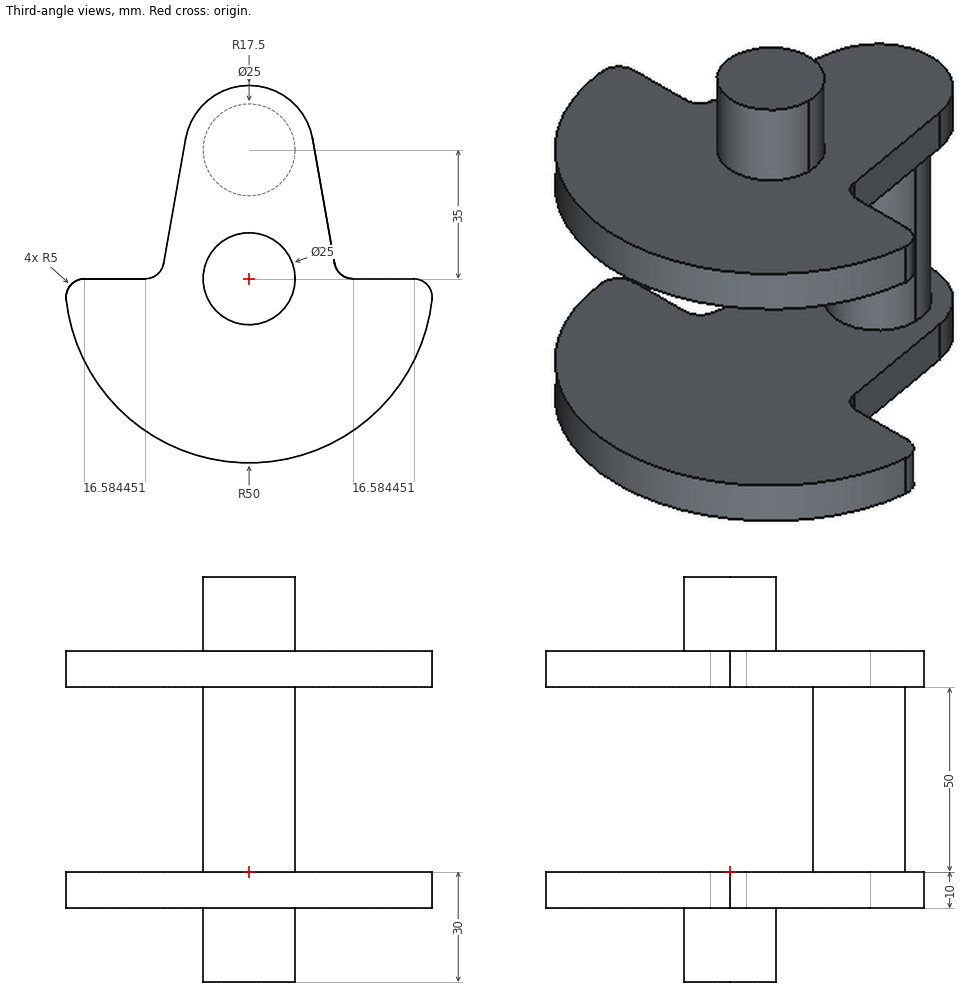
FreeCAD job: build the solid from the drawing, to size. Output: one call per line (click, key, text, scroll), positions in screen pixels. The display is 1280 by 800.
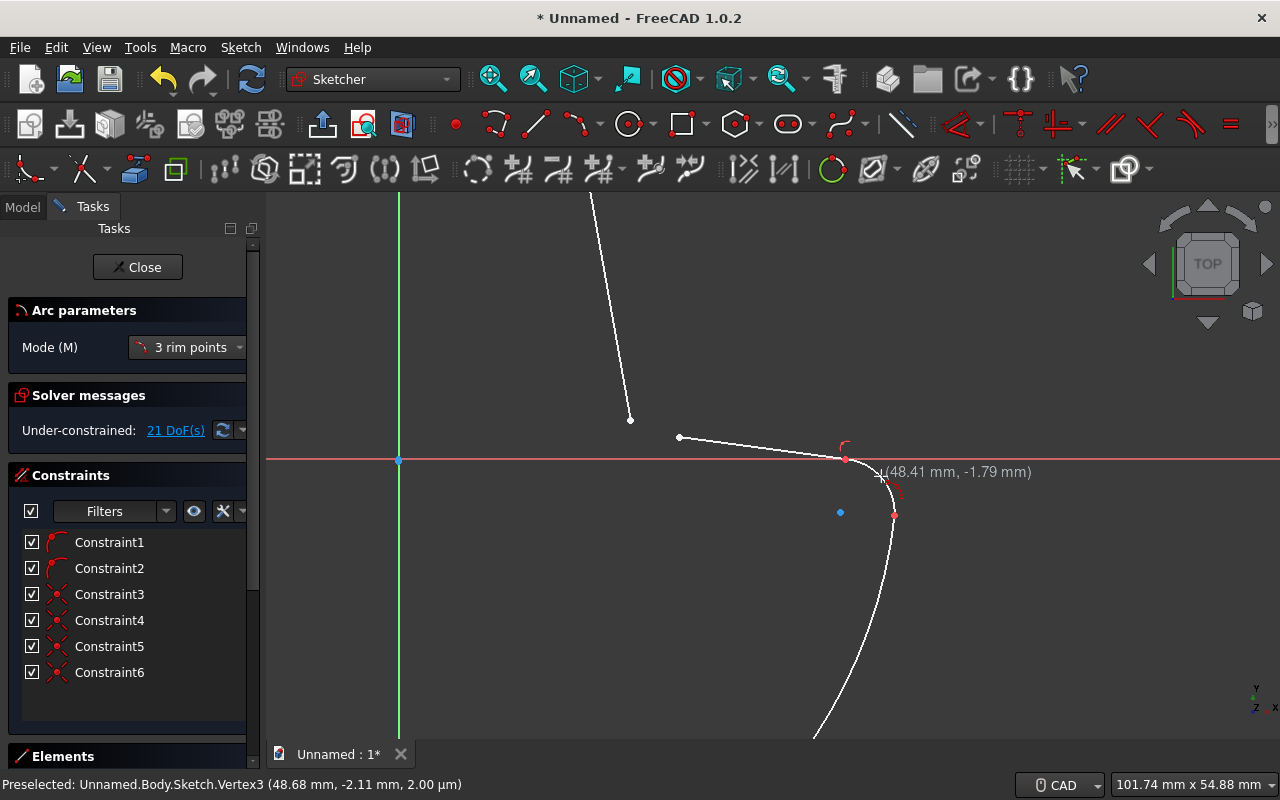
click(680, 437)
click(631, 421)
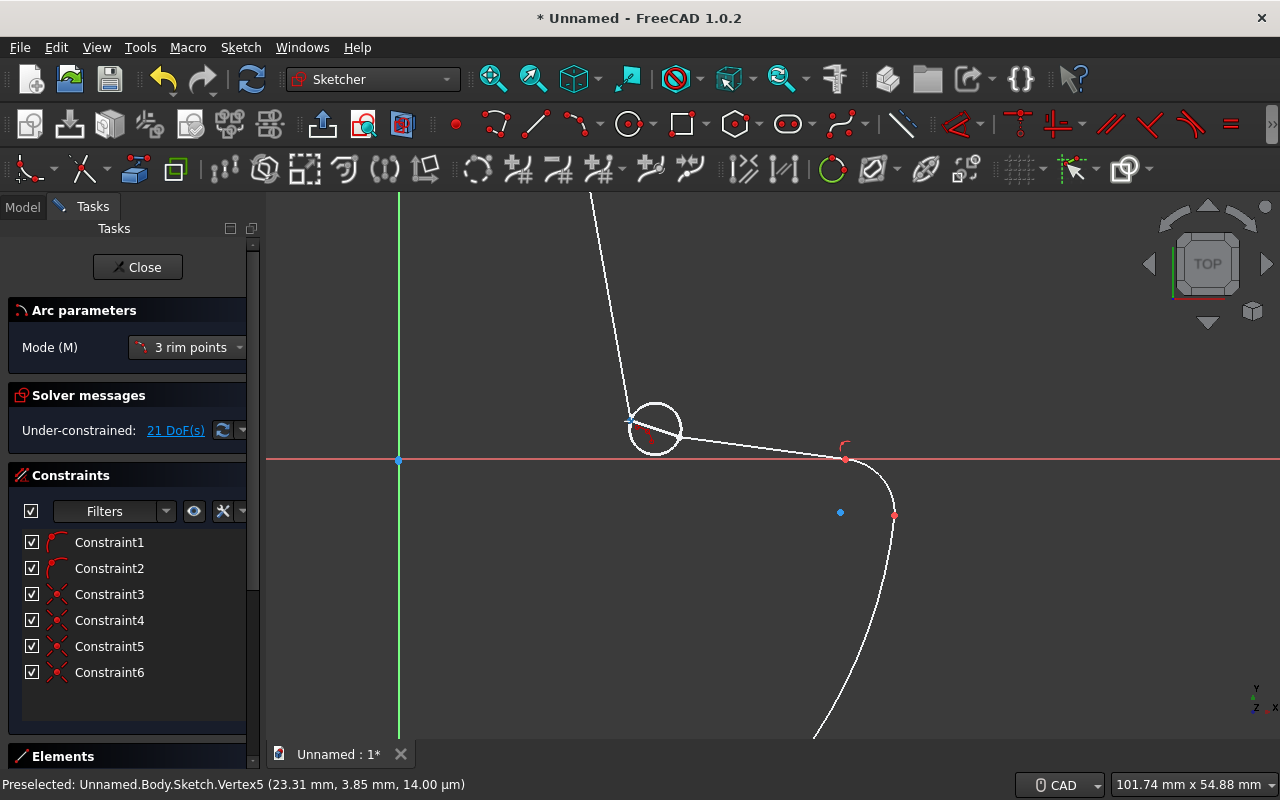
scroll(647, 447, up, 2)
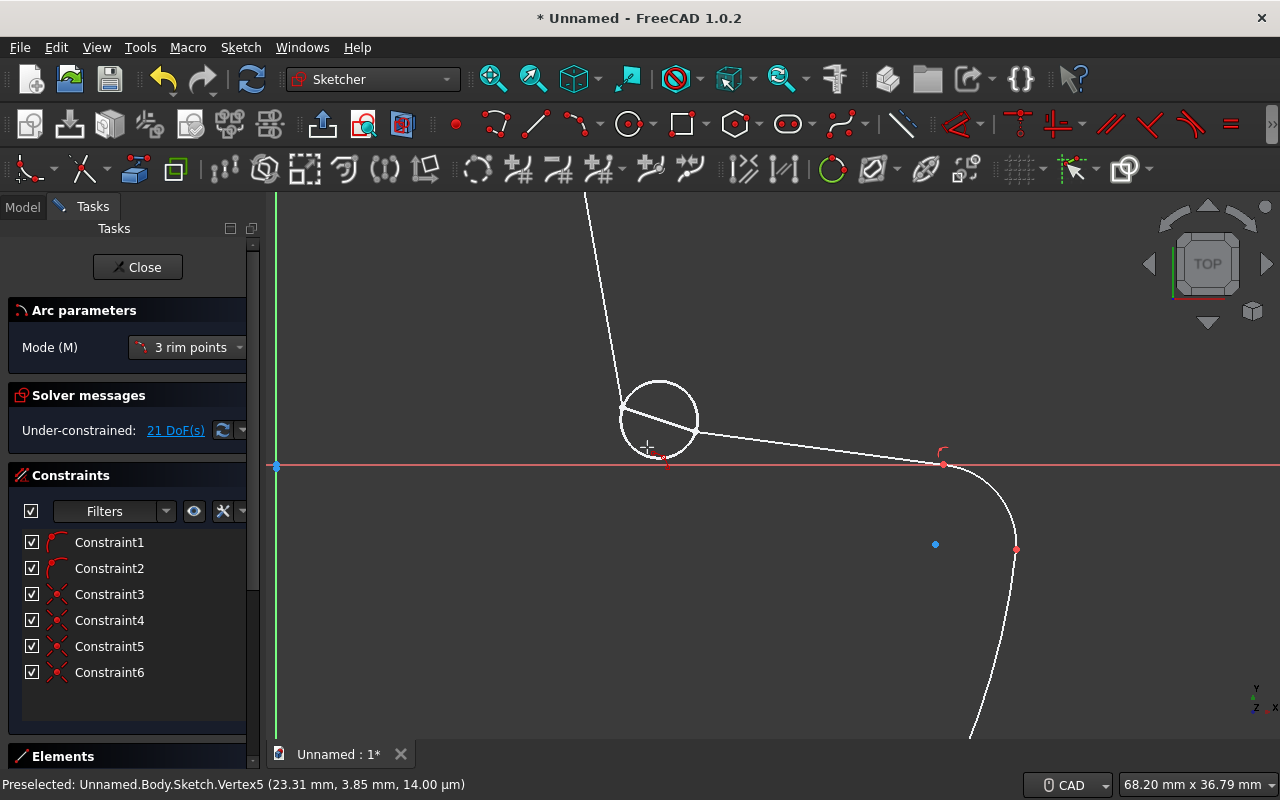
click(647, 447)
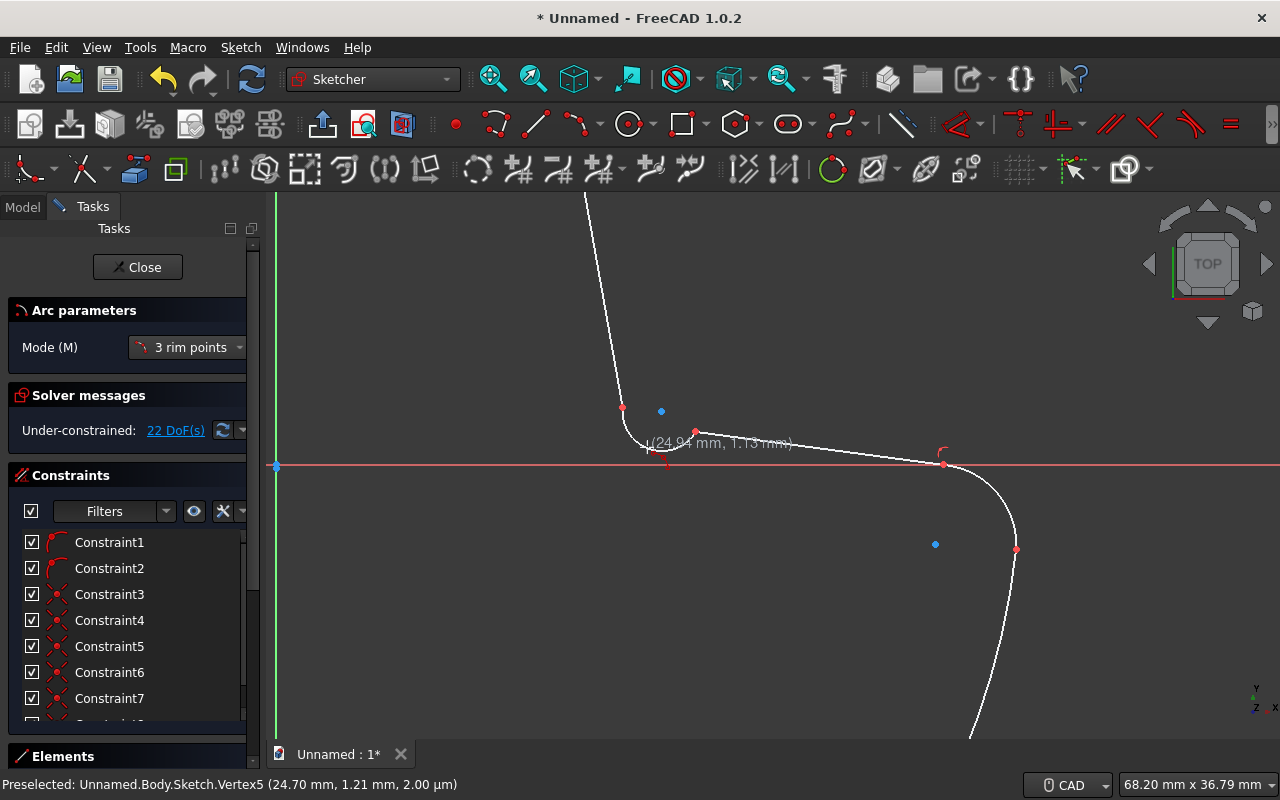
scroll(845, 472, down, 7)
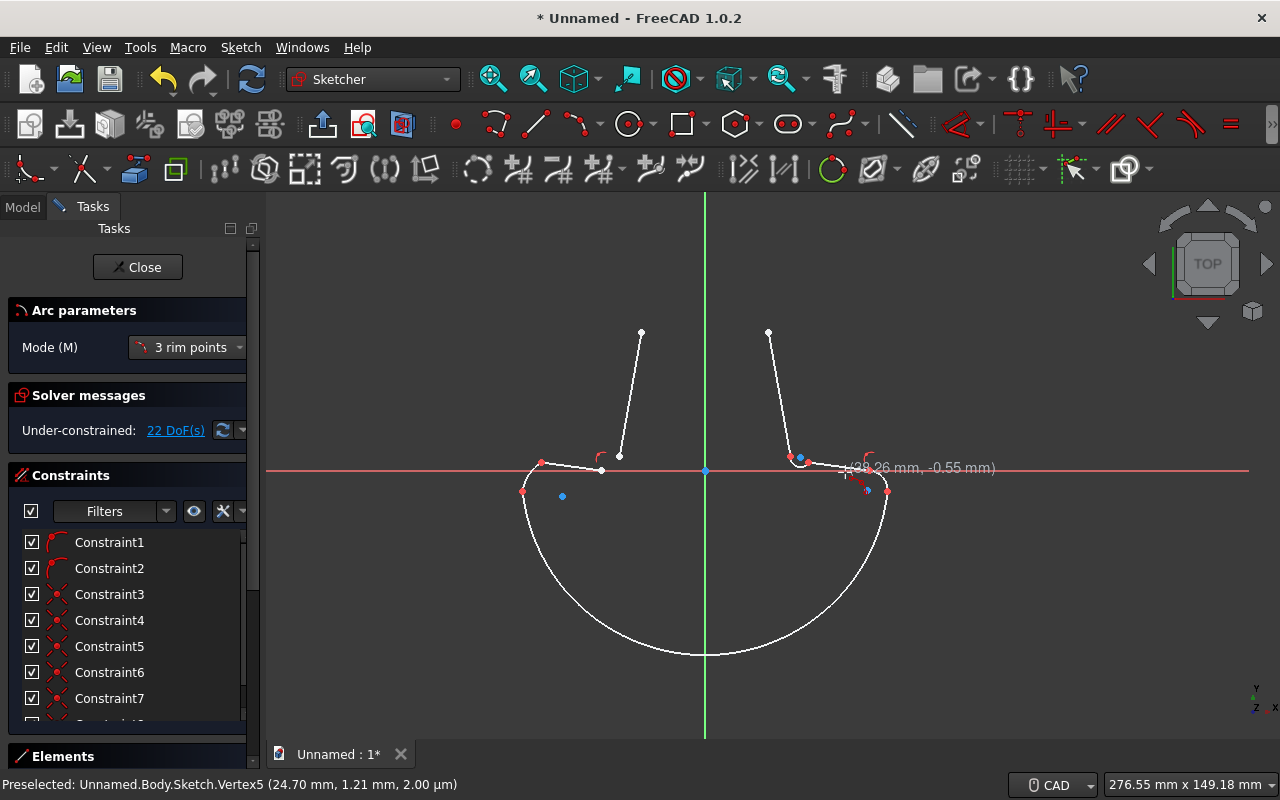
click(769, 333)
click(642, 333)
click(723, 281)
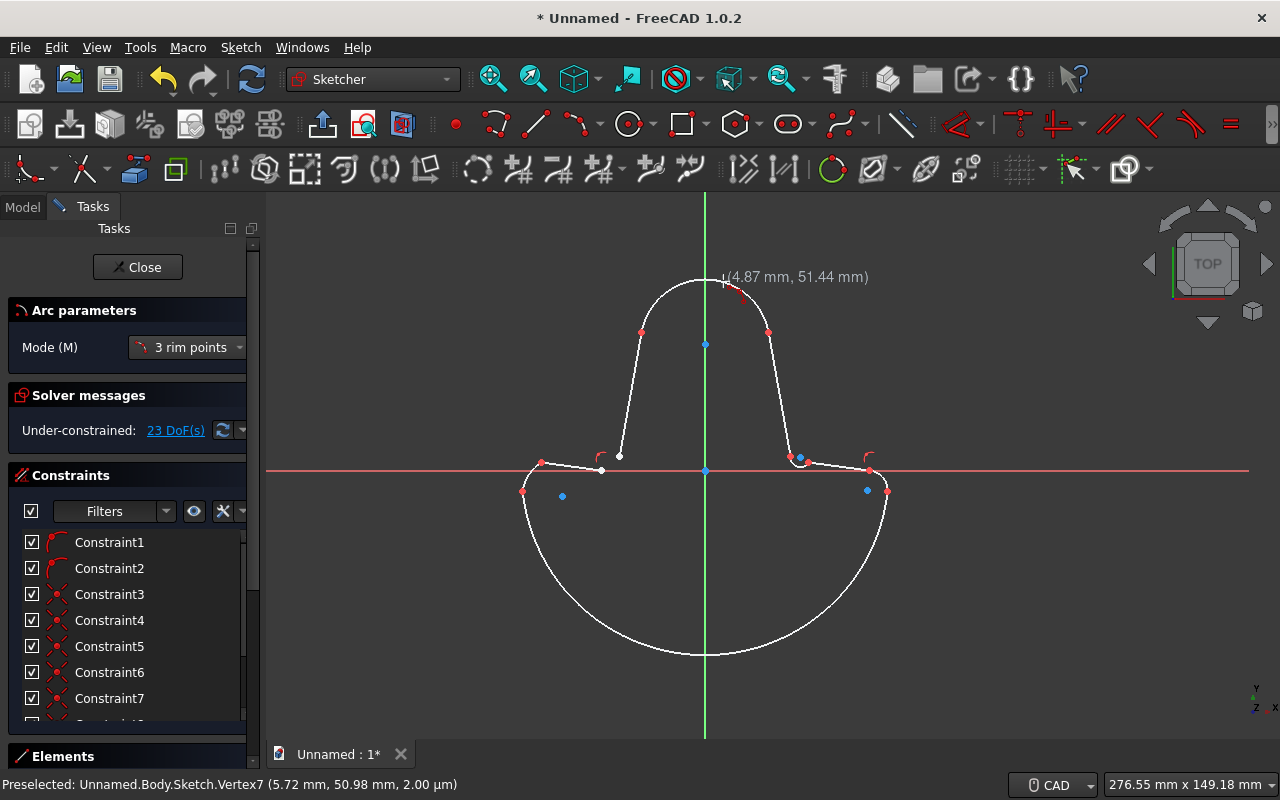
click(620, 457)
click(602, 471)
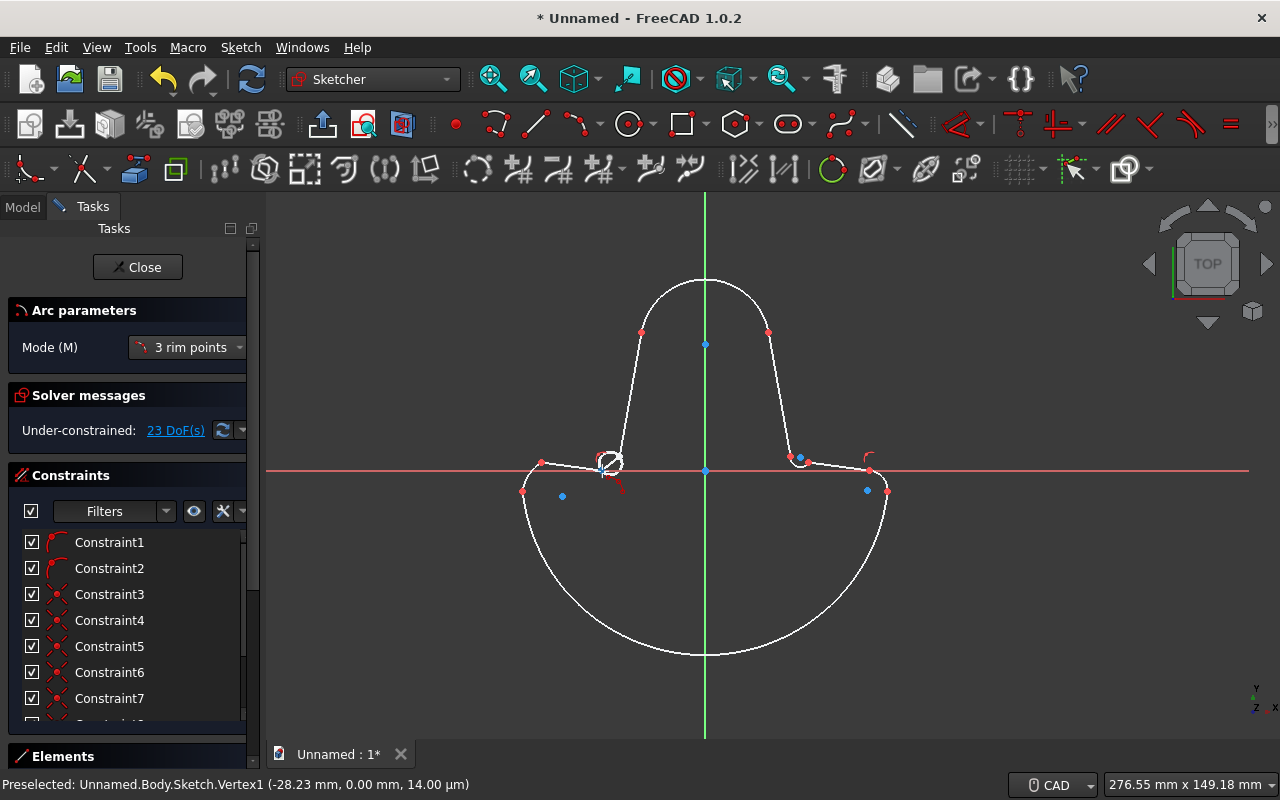
scroll(614, 466, up, 7)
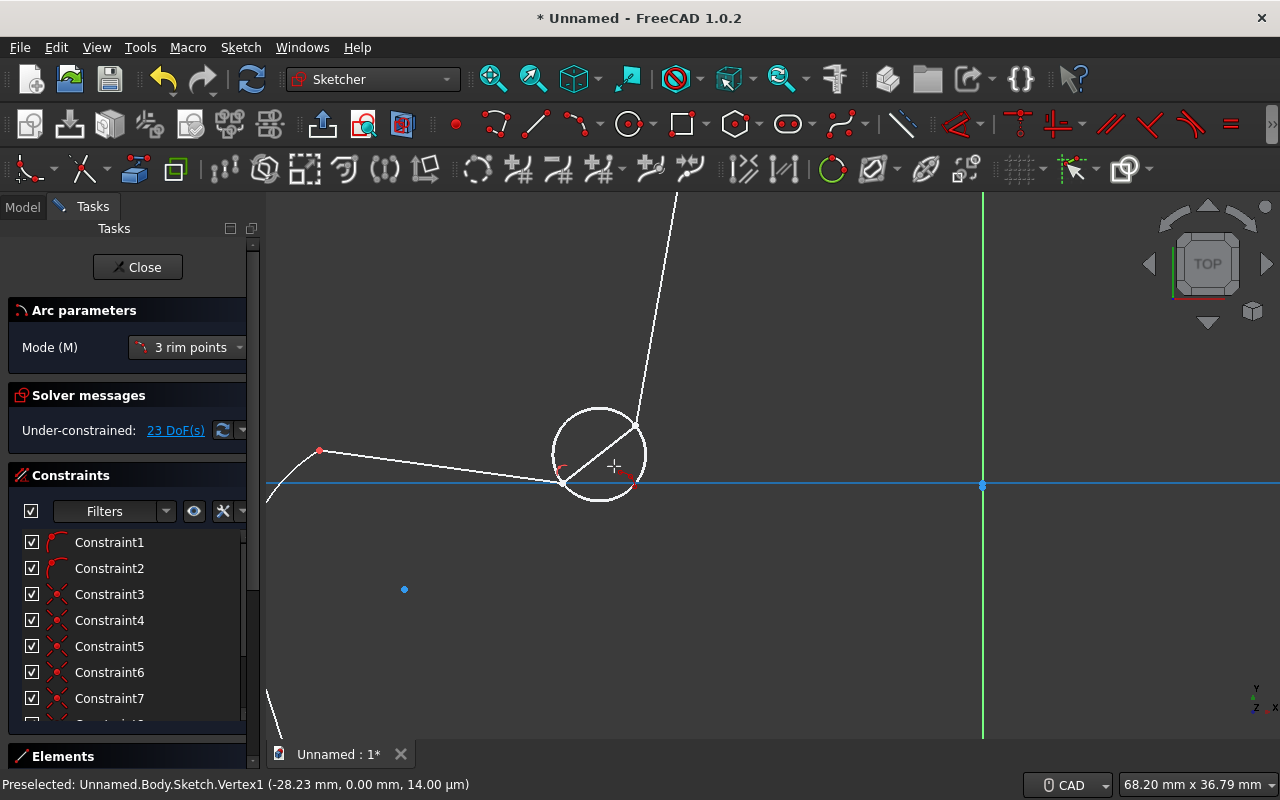
click(612, 466)
key(Escape)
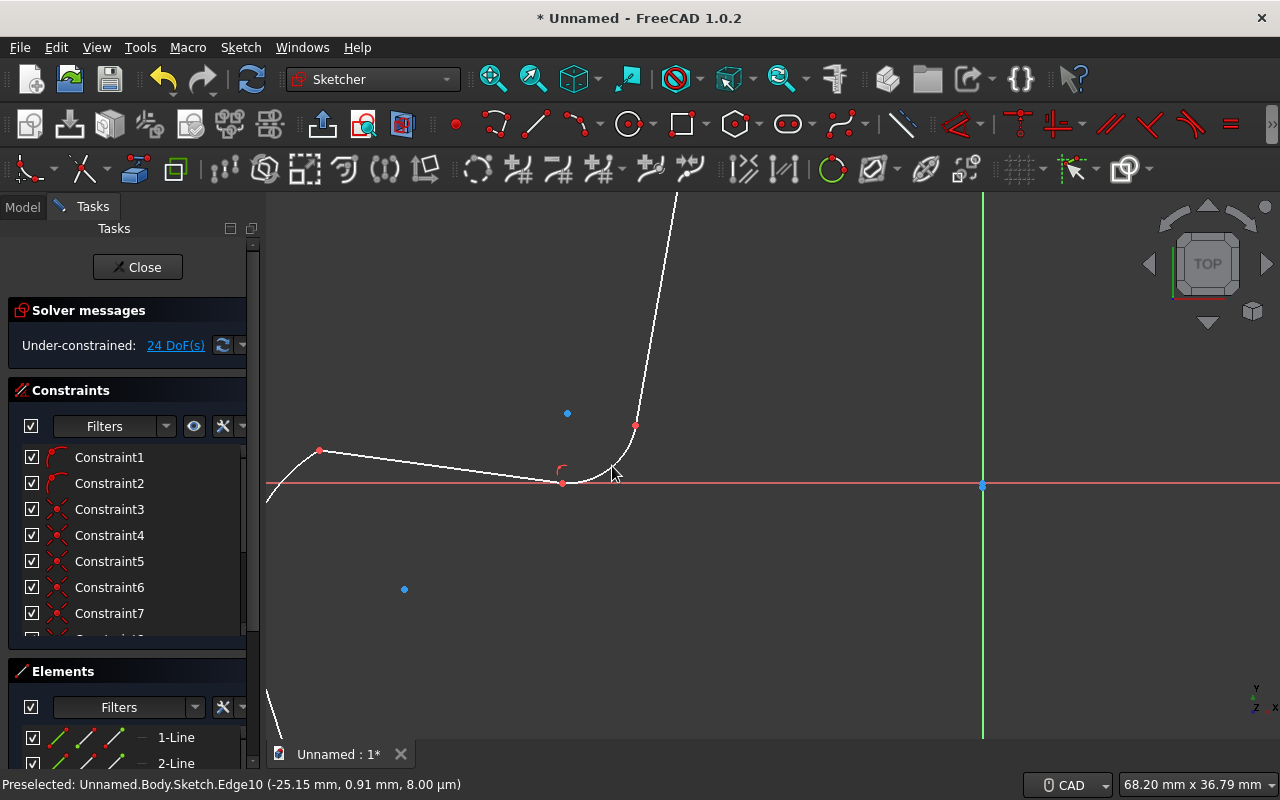
scroll(490, 473, up, 2)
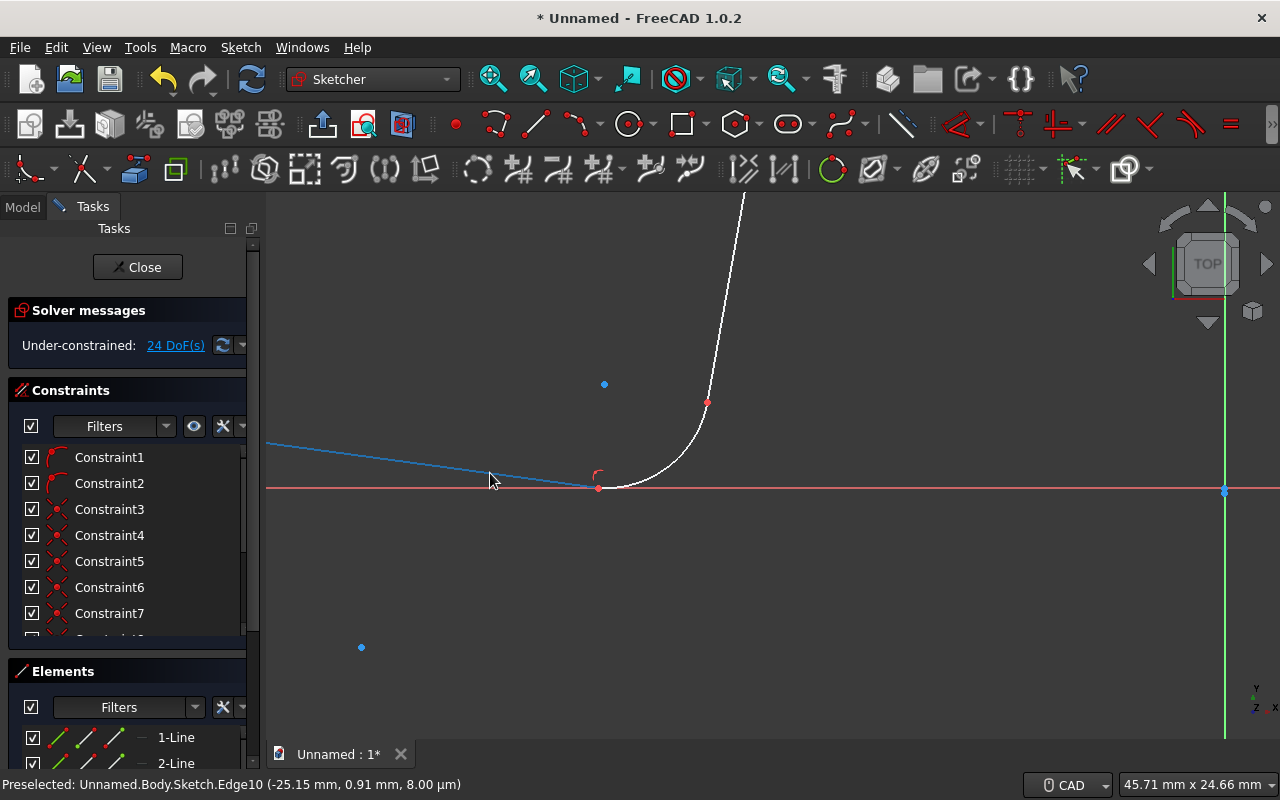
click(490, 473)